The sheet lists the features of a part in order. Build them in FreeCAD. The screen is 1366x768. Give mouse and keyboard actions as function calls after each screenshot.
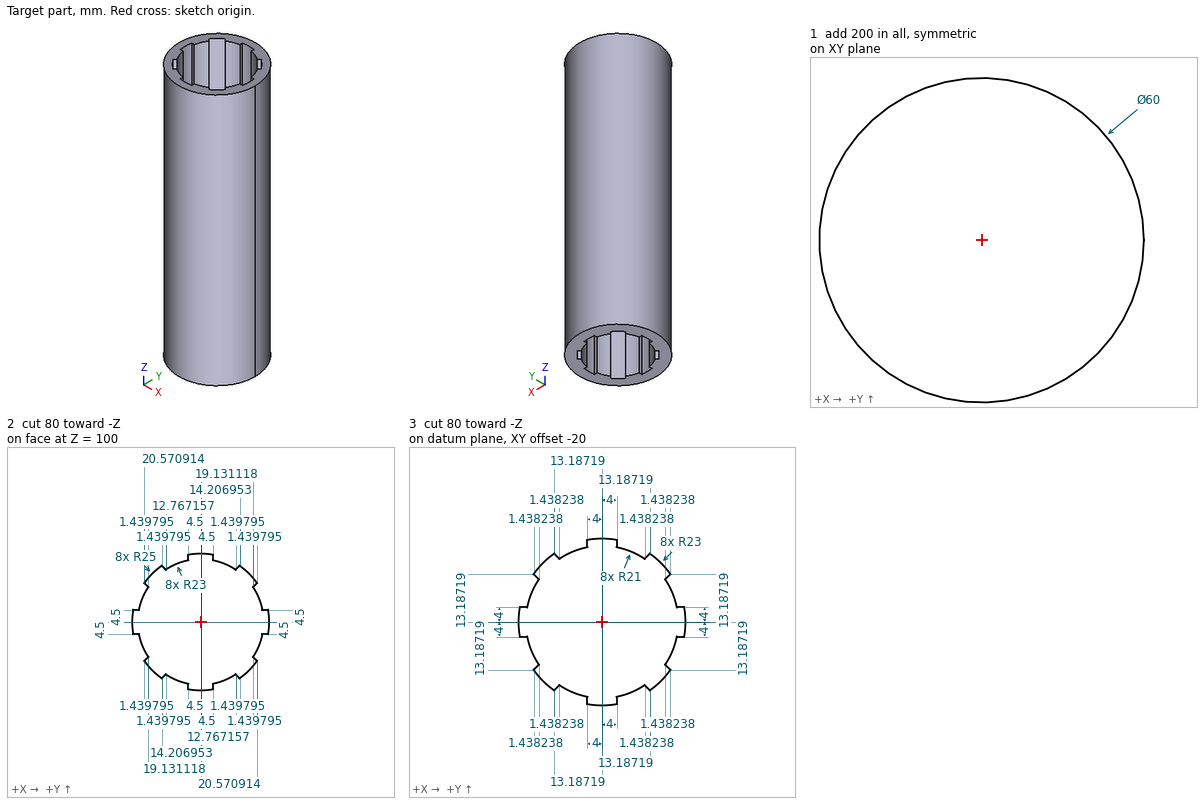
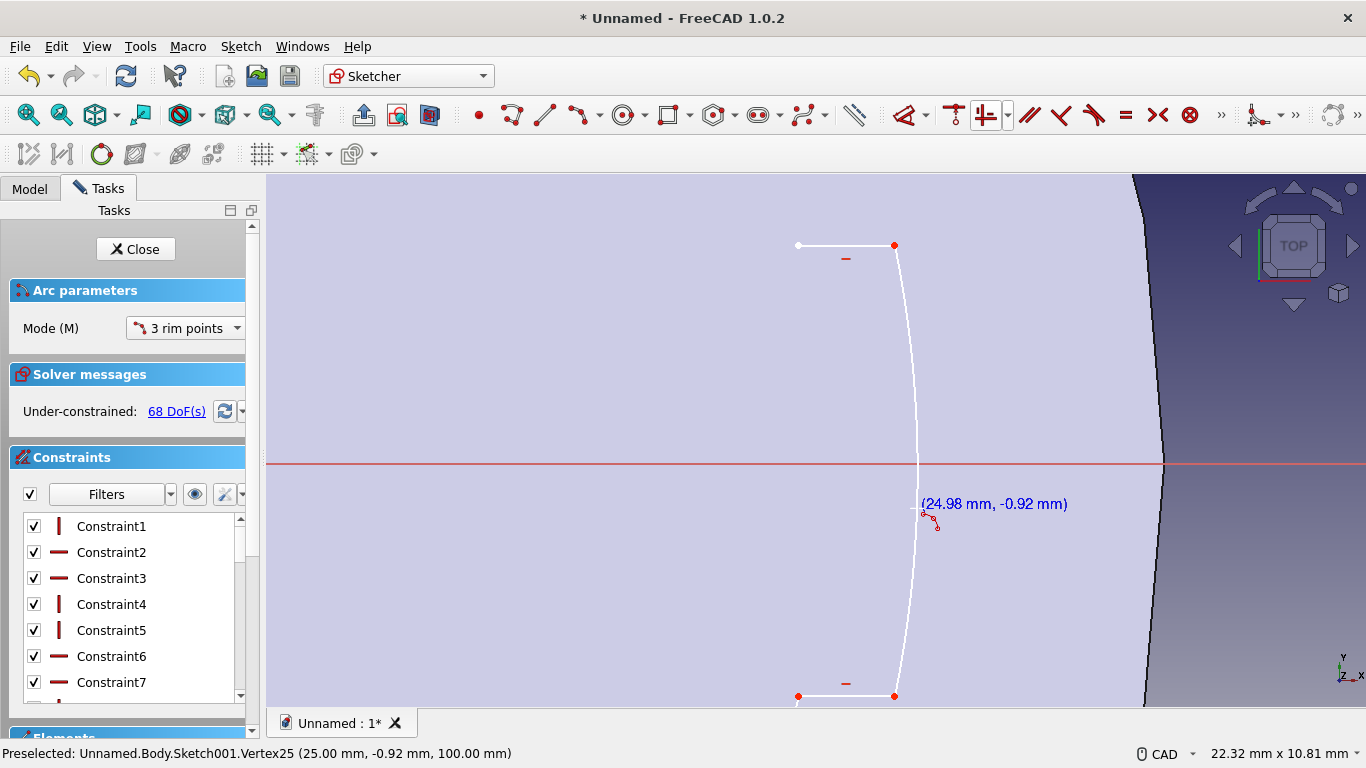
scroll(914, 437, down, 10)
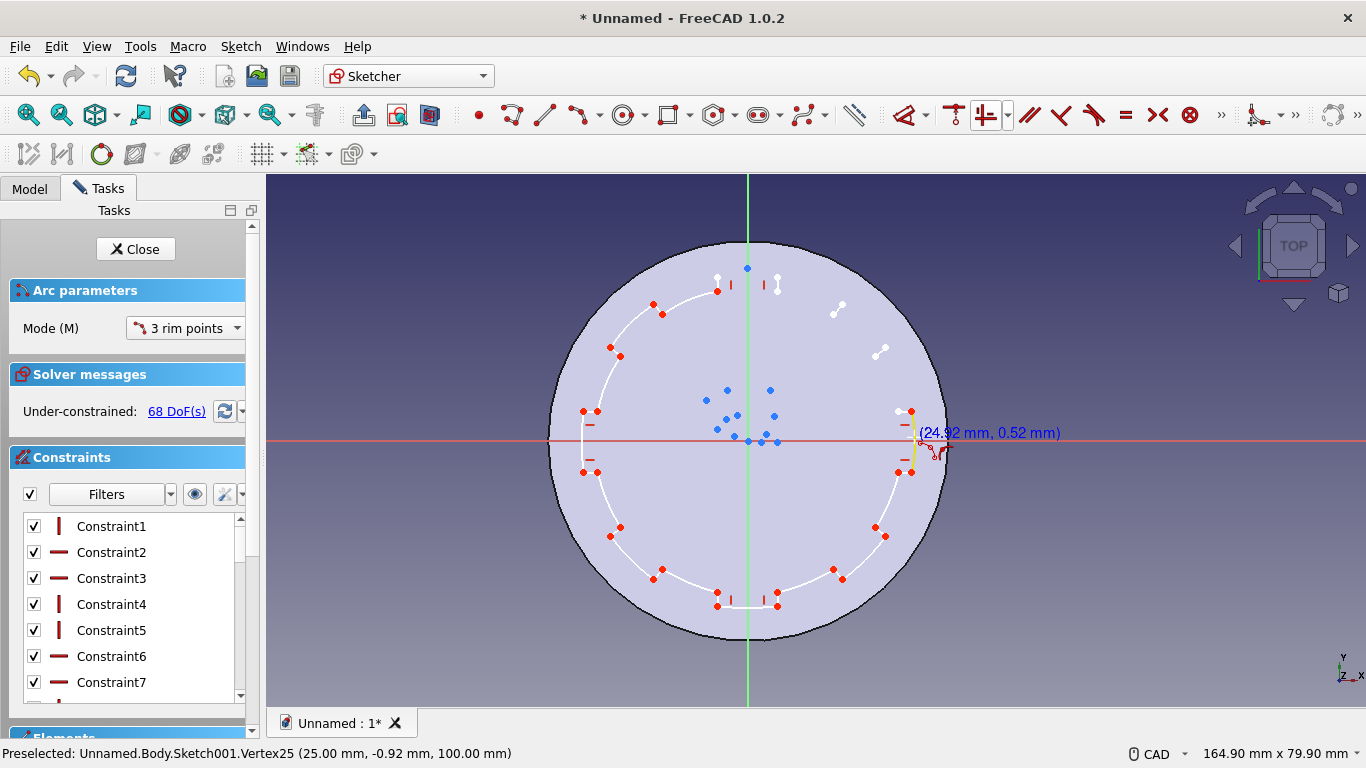
scroll(899, 411, up, 5)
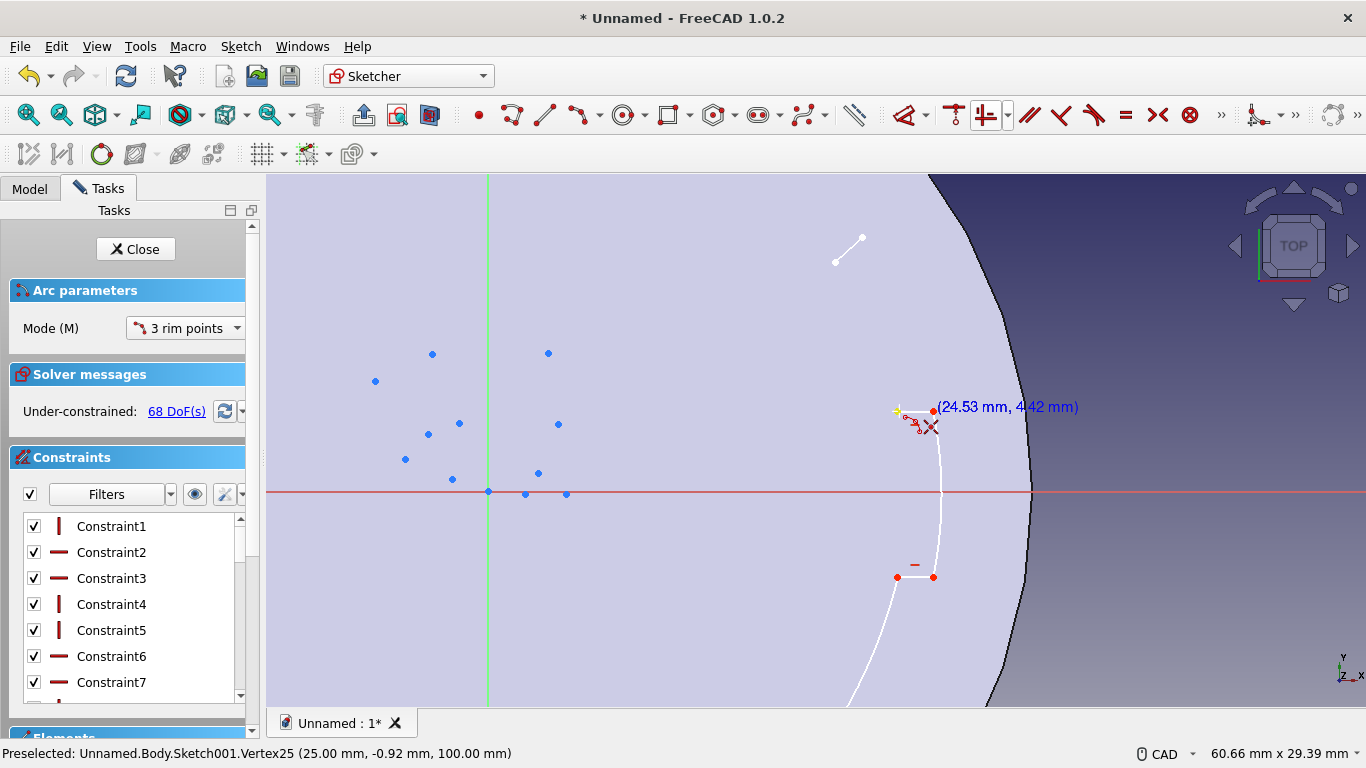
click(898, 412)
click(835, 262)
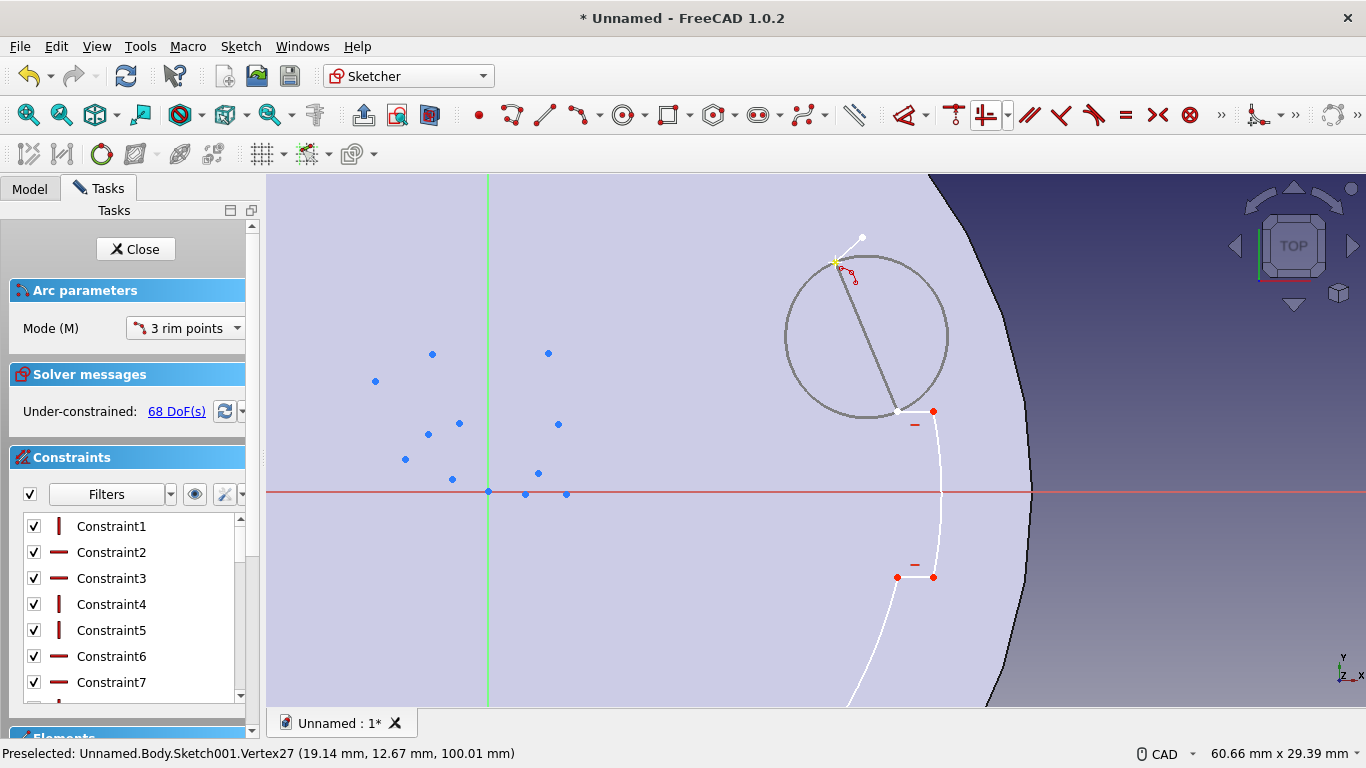
scroll(874, 332, up, 4)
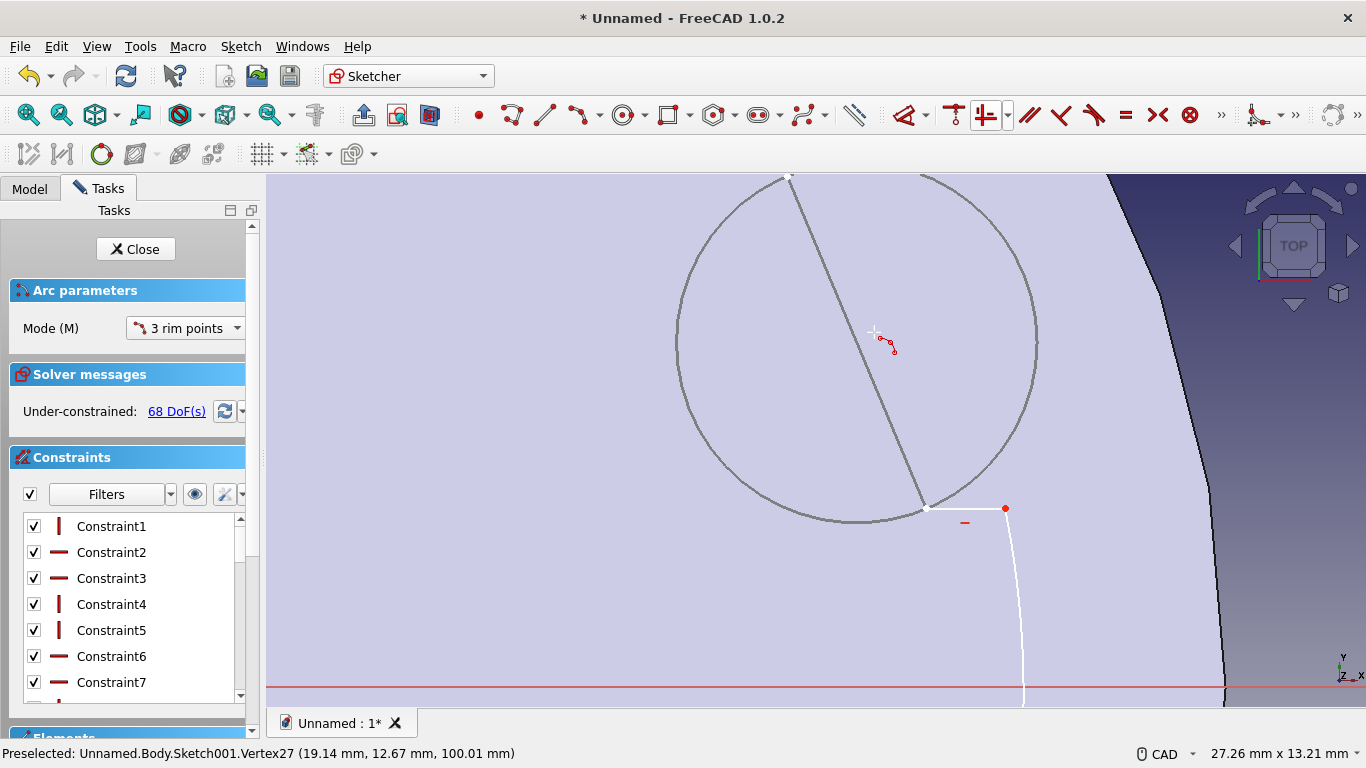
click(872, 332)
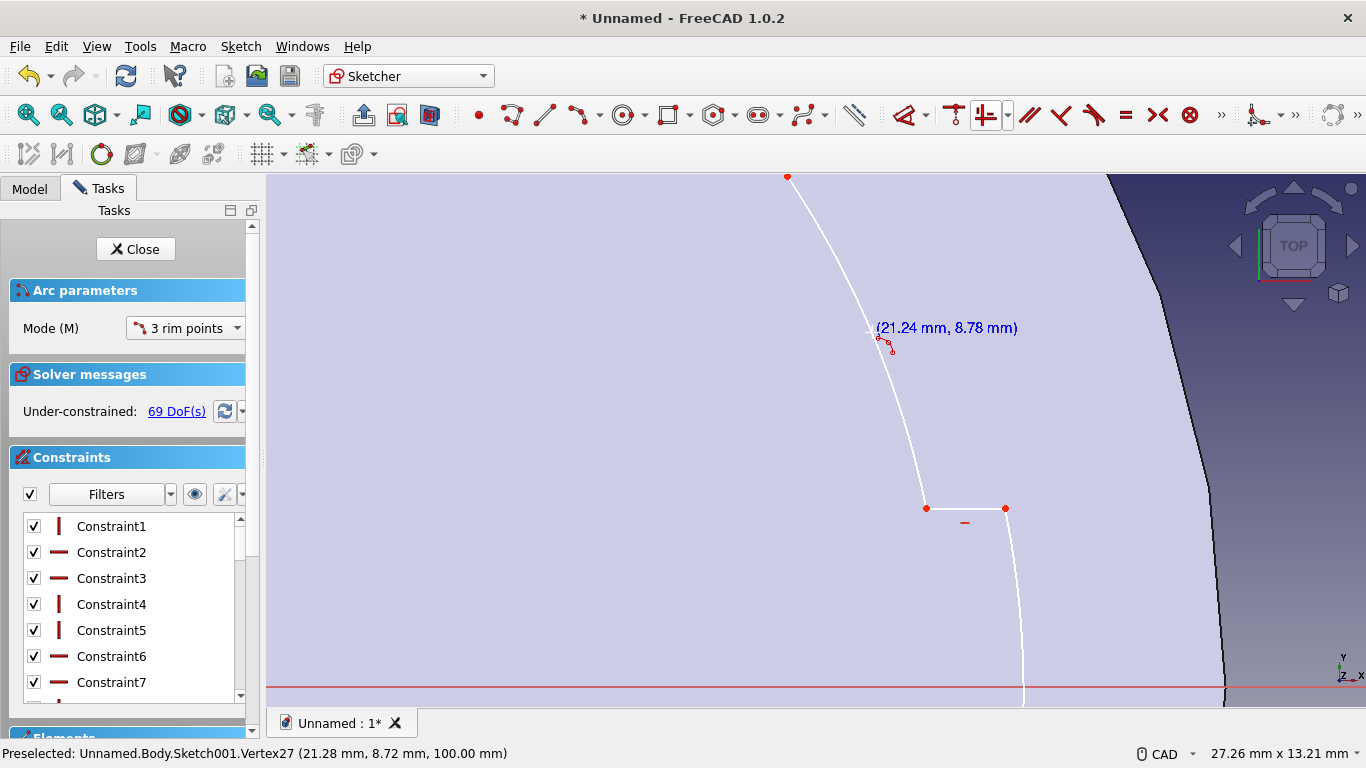
scroll(893, 392, down, 9)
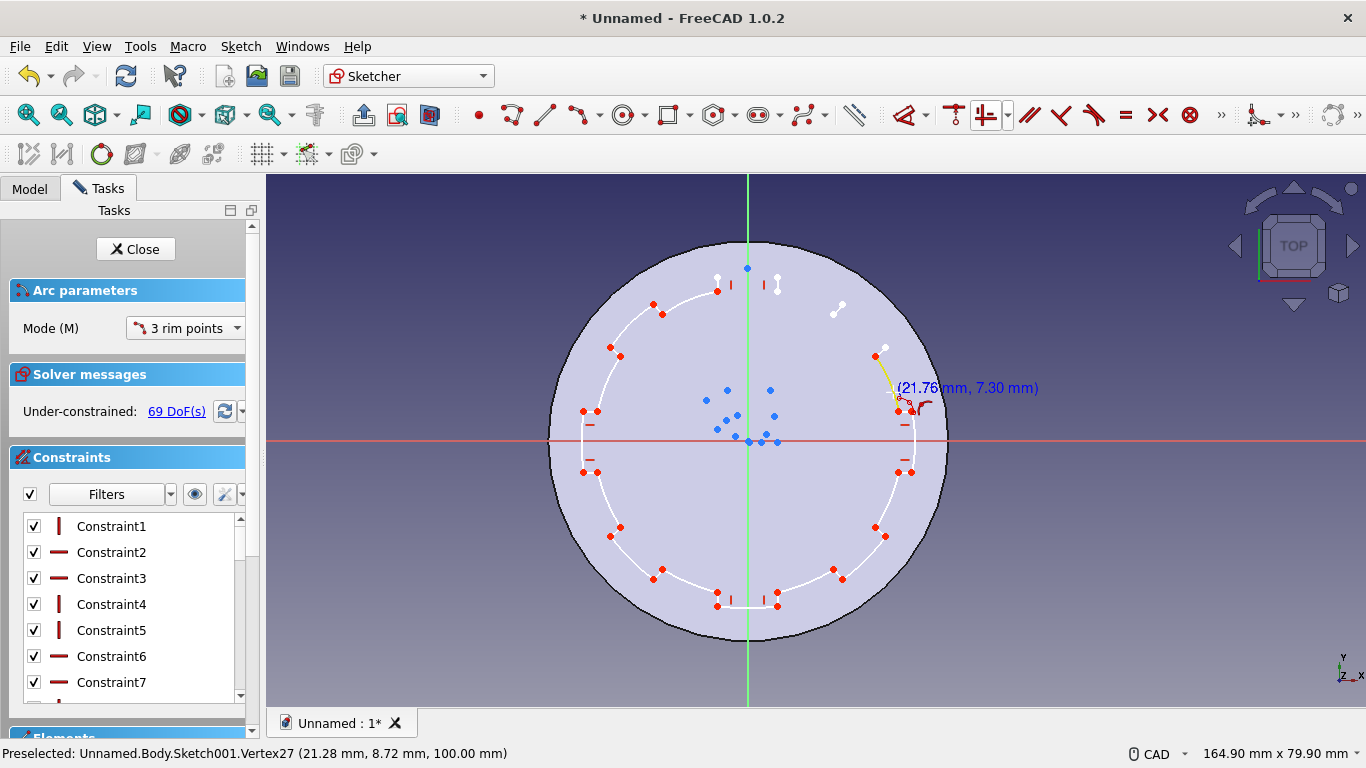
scroll(886, 346, up, 5)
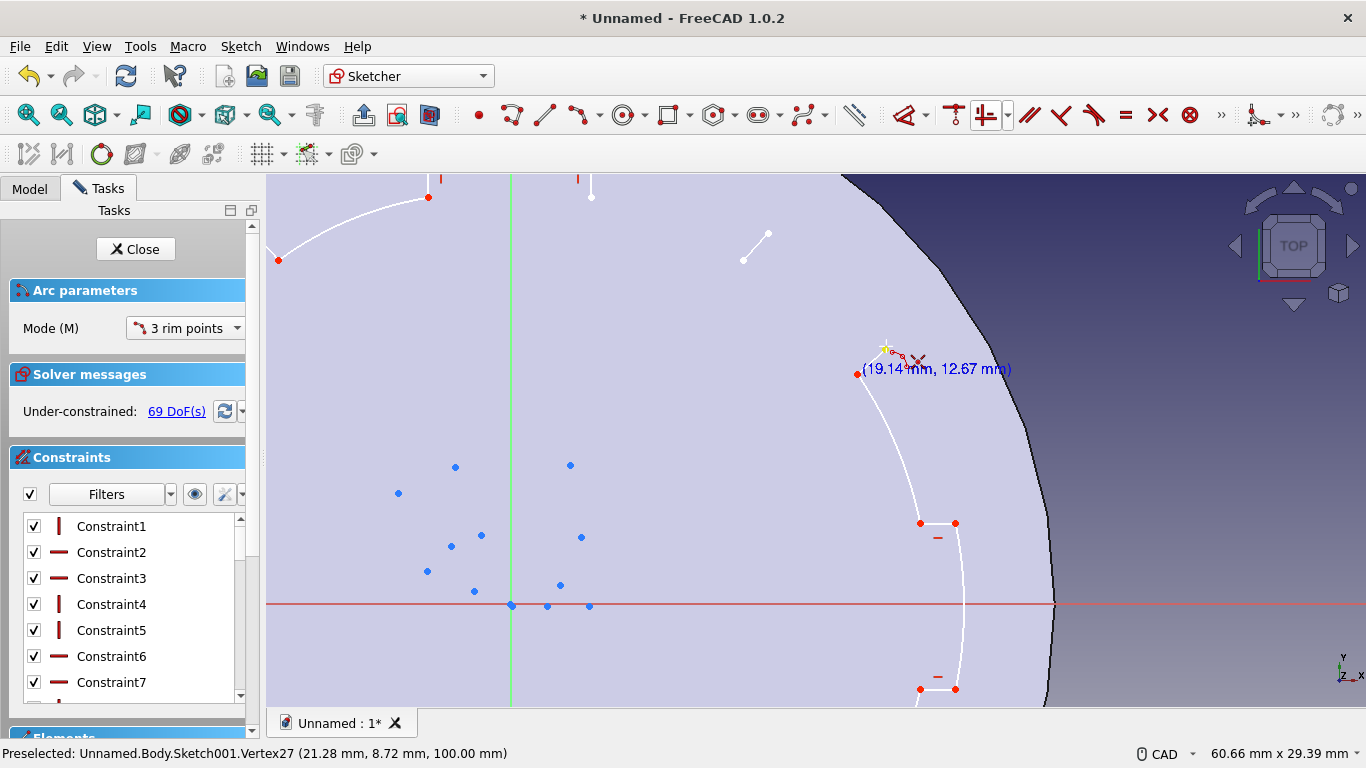
click(885, 350)
click(768, 233)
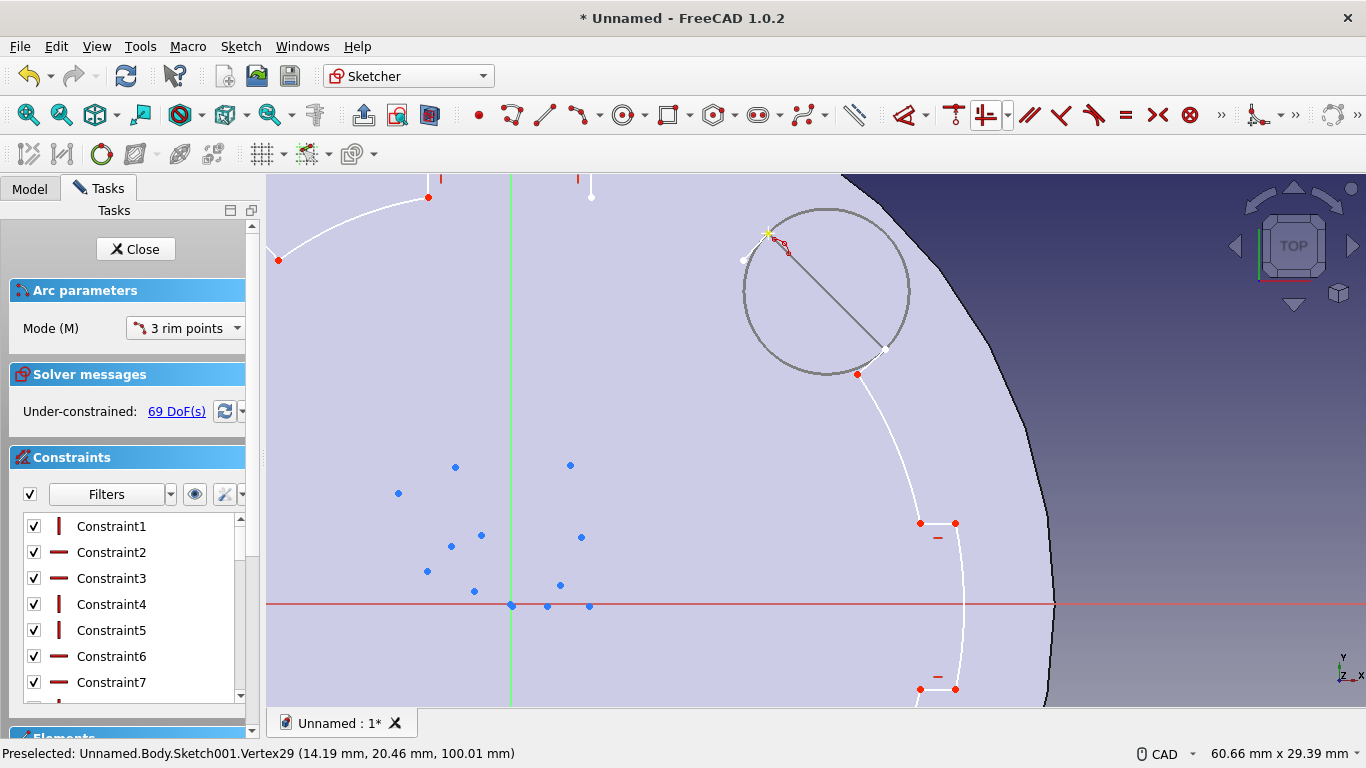
scroll(831, 284, up, 4)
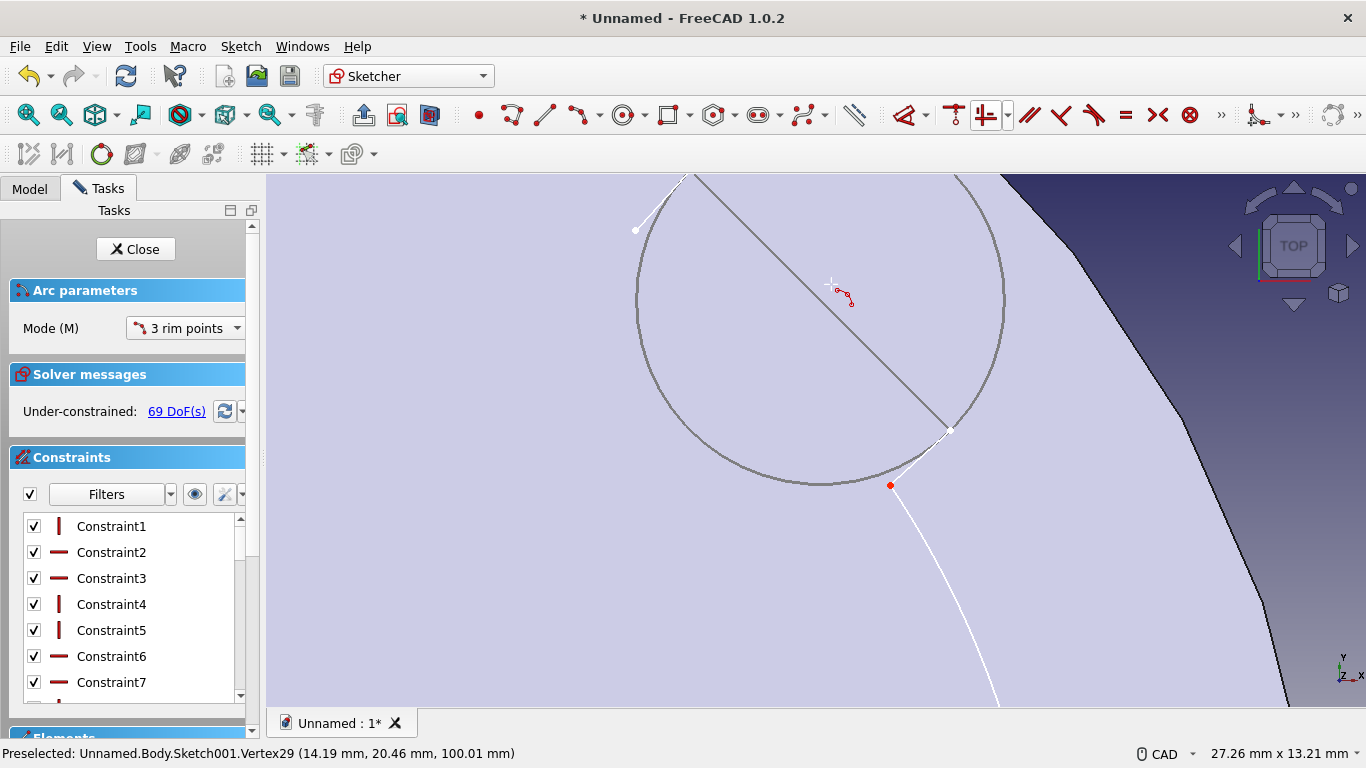
click(831, 283)